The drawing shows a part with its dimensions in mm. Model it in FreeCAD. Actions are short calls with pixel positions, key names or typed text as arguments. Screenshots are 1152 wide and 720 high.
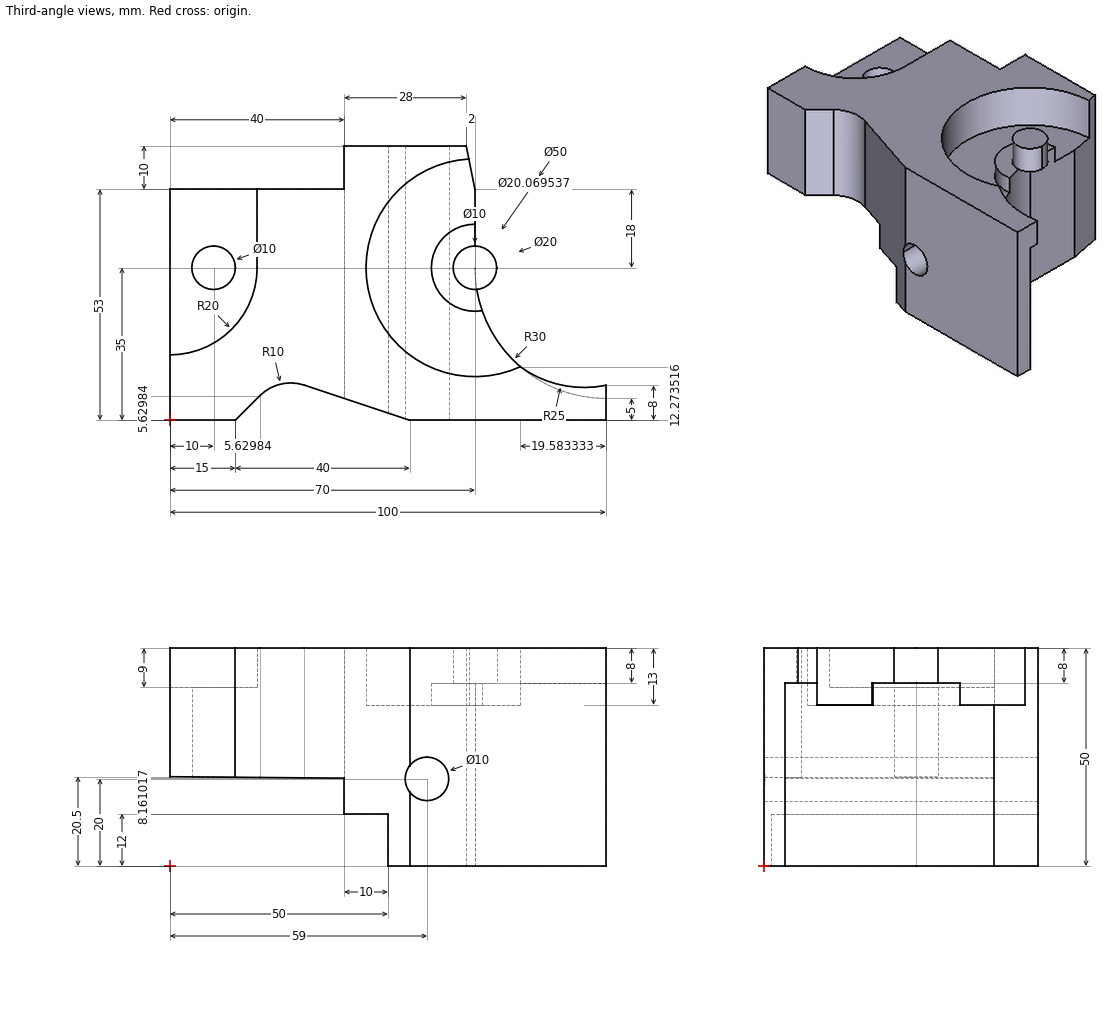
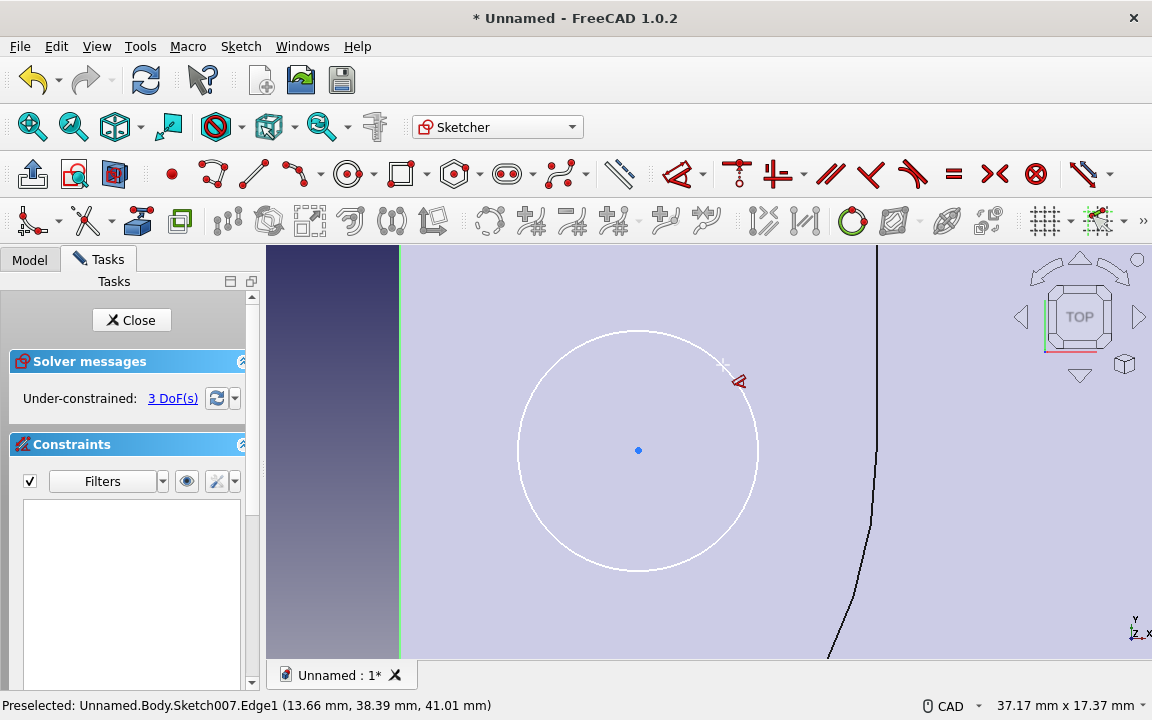
click(723, 366)
click(746, 343)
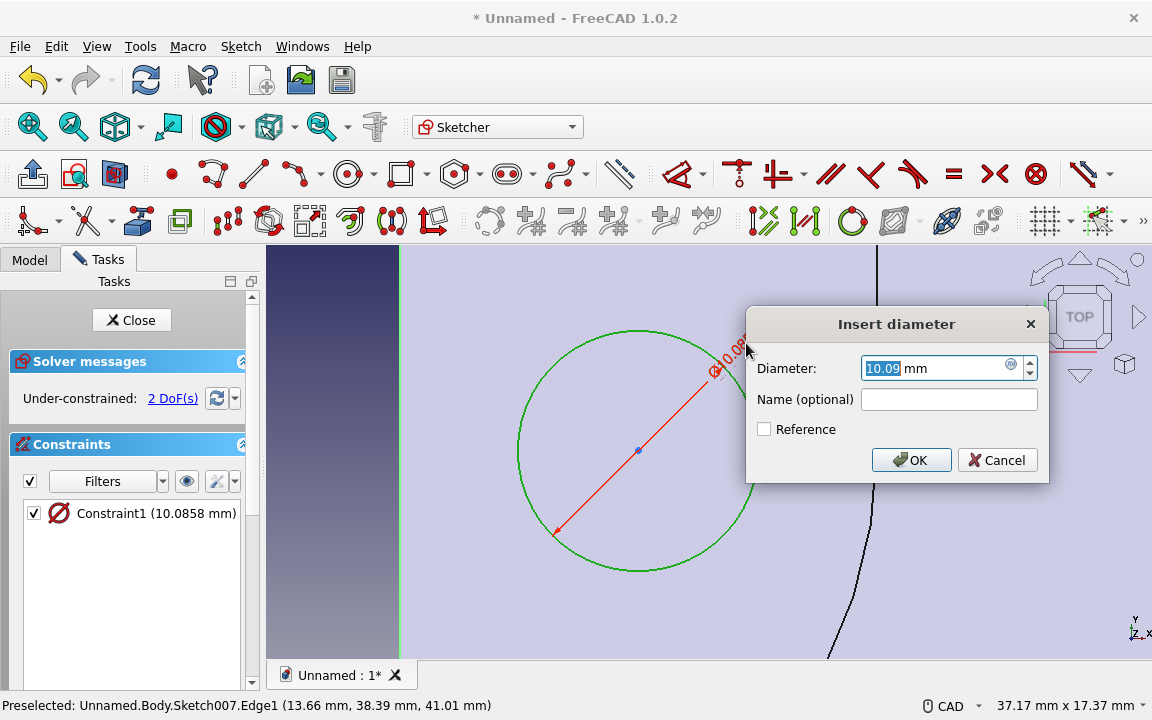
text(10)
key(Return)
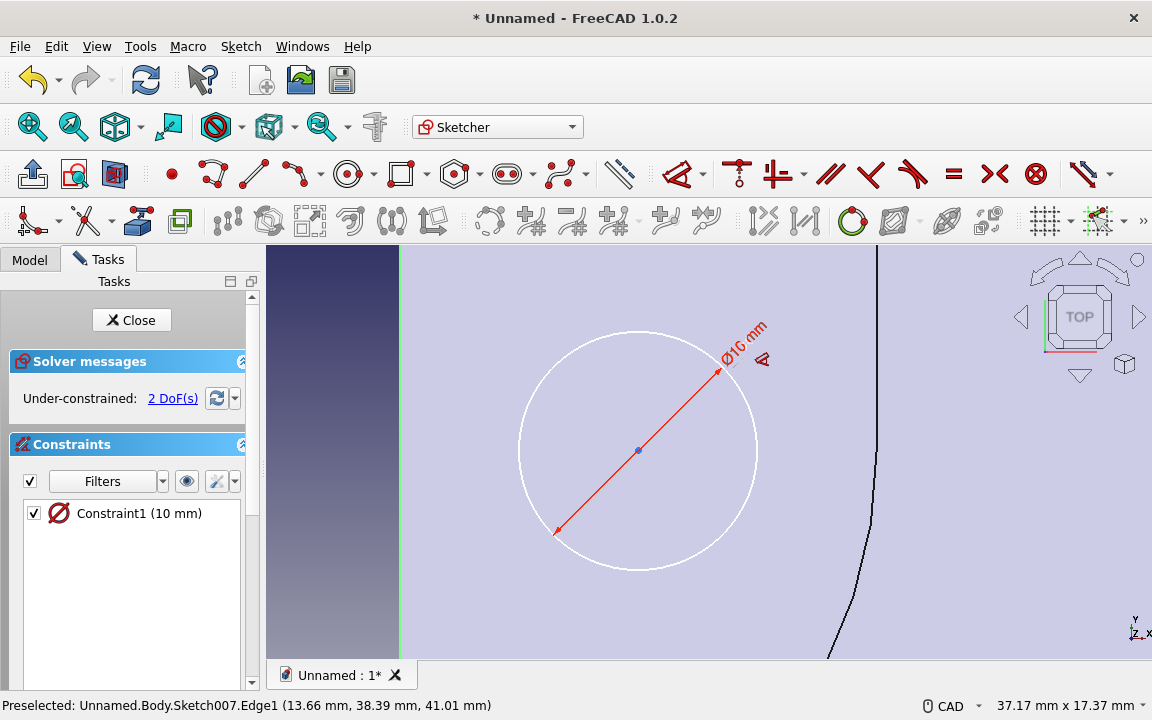
click(638, 451)
click(464, 417)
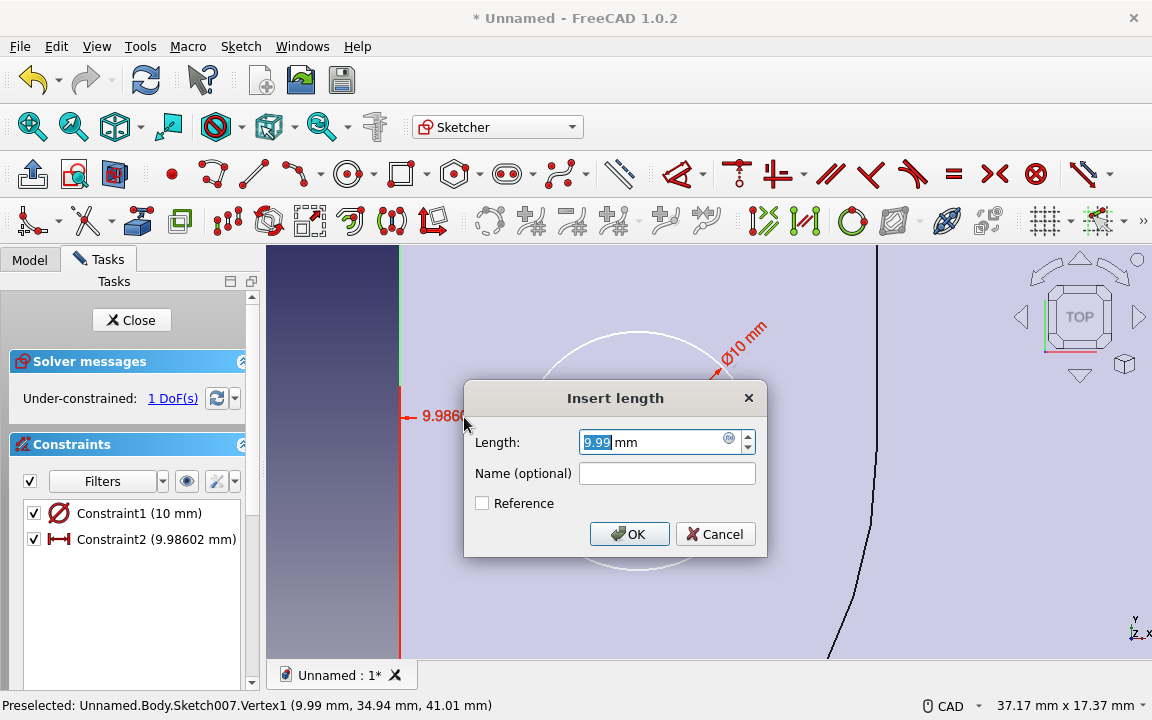
text(10)
key(Return)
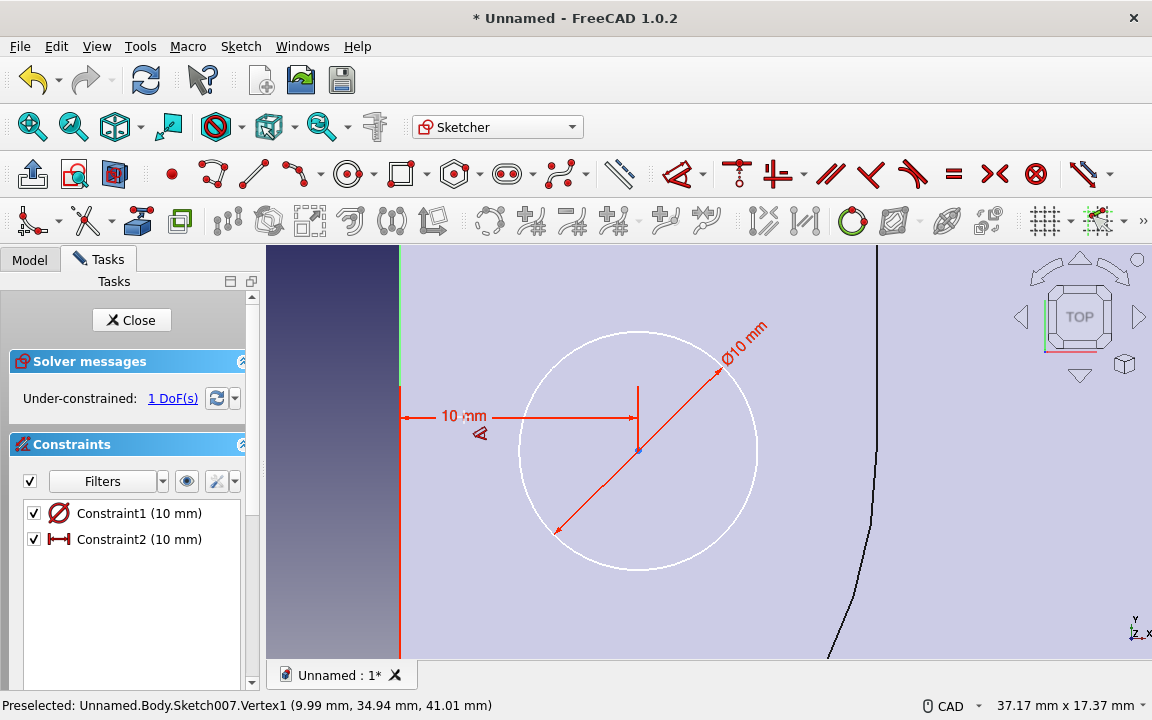
click(638, 451)
click(366, 541)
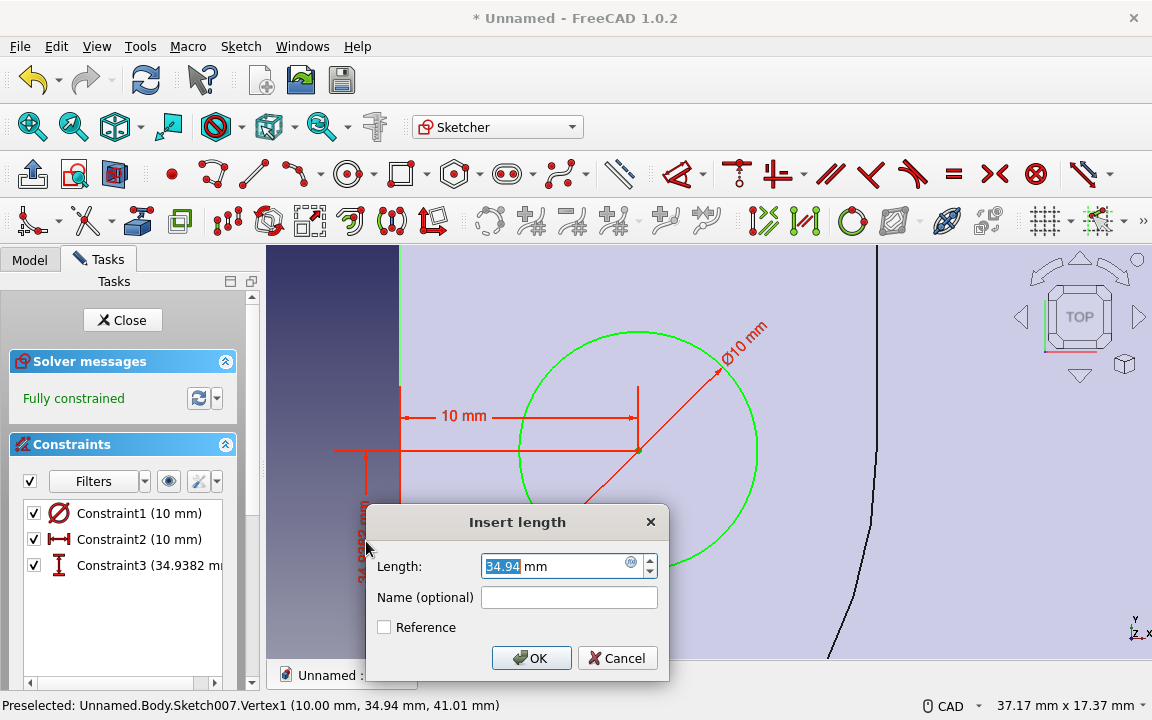
text(35)
key(Return)
key(Escape)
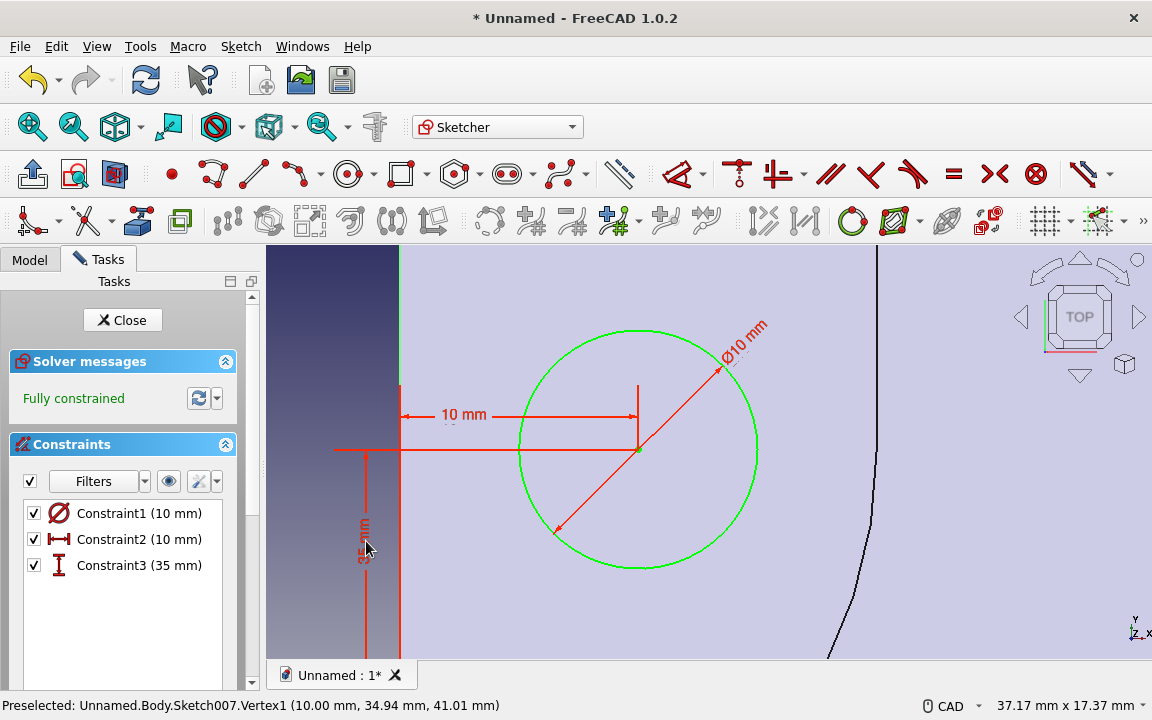
click(123, 320)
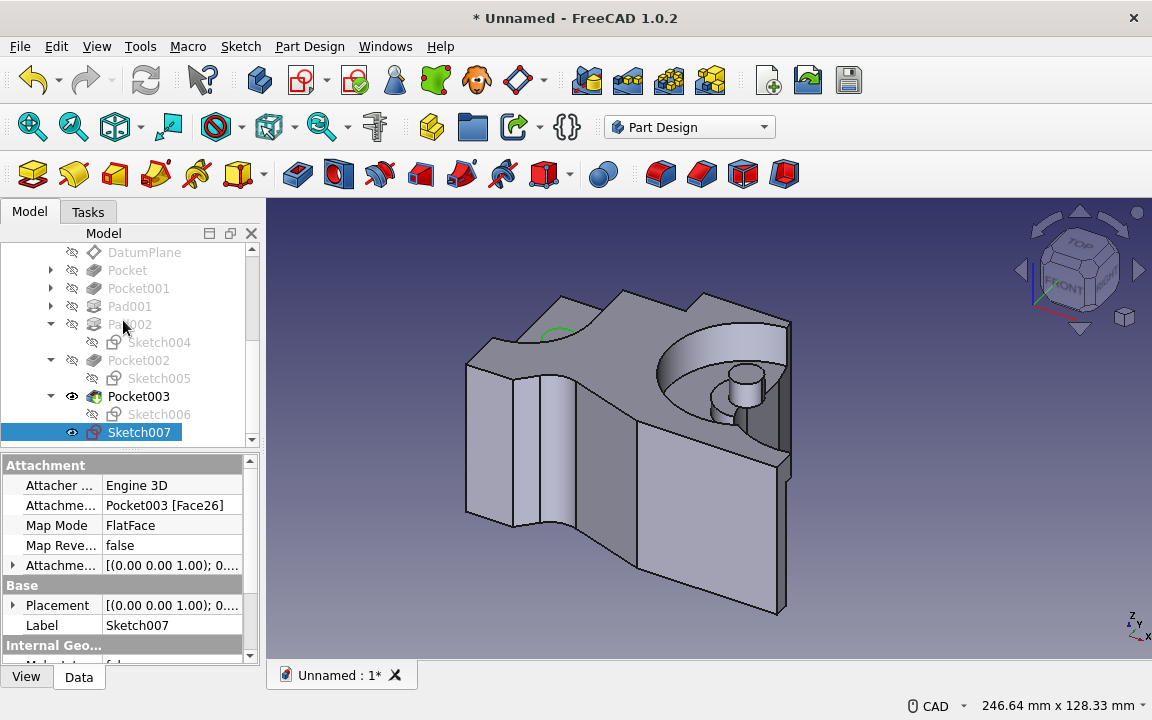
click(298, 174)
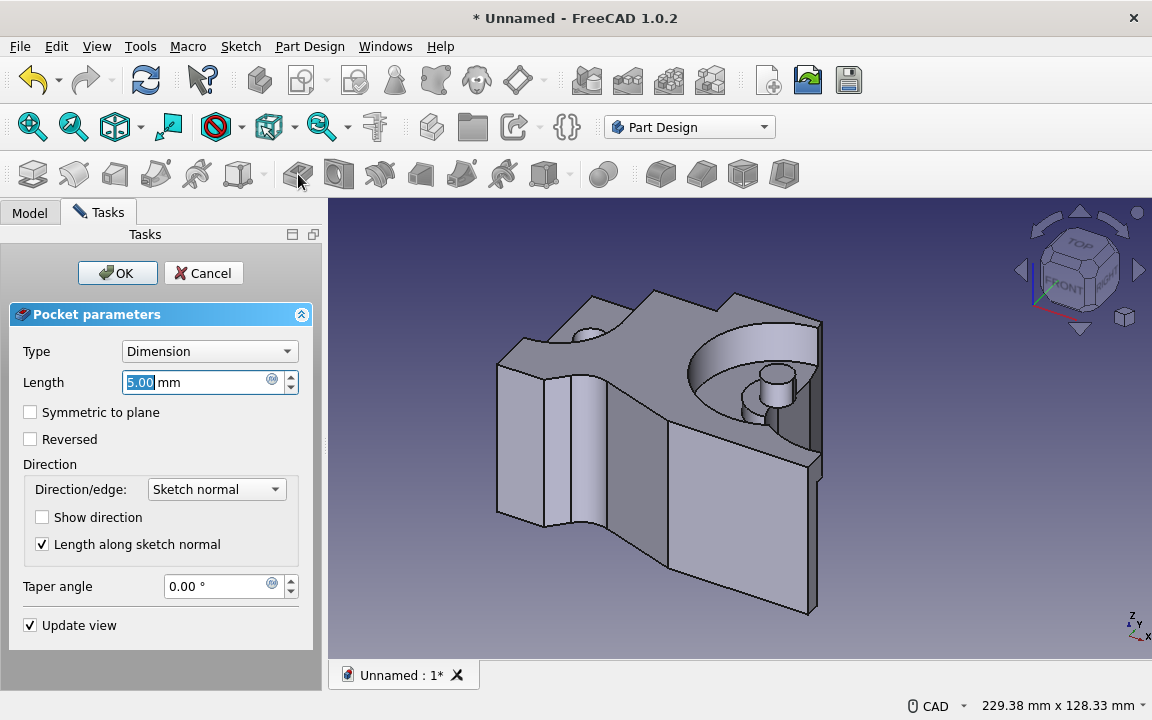
click(210, 352)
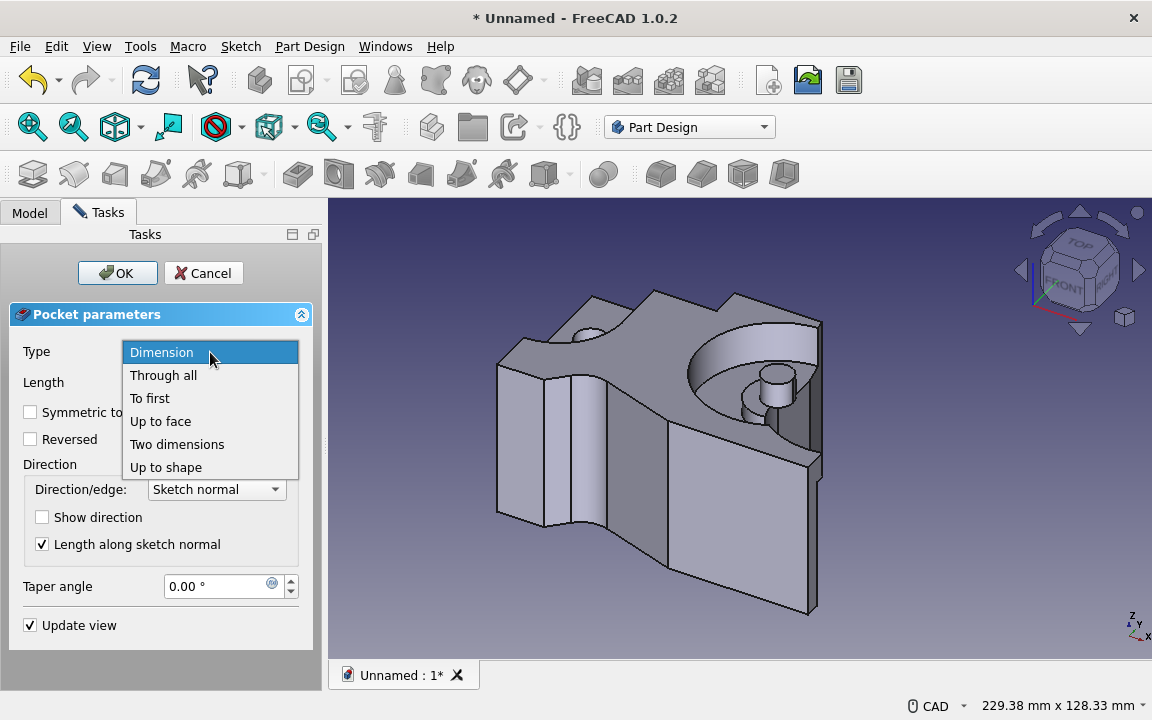
click(208, 376)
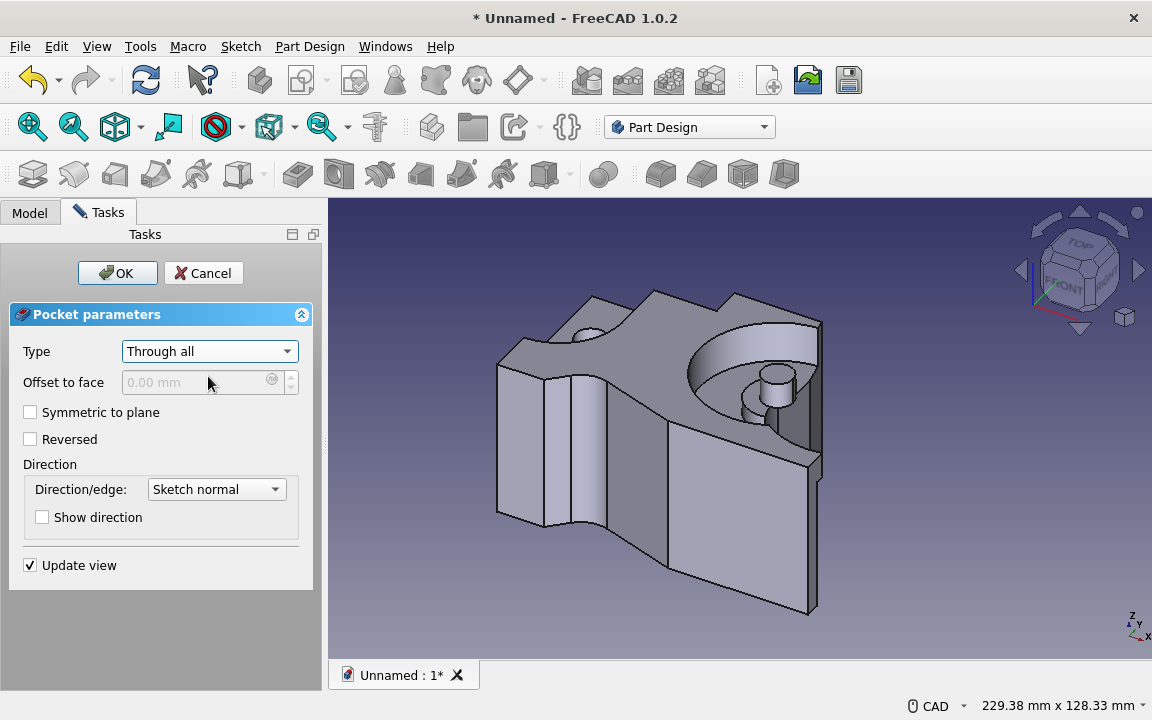
click(118, 273)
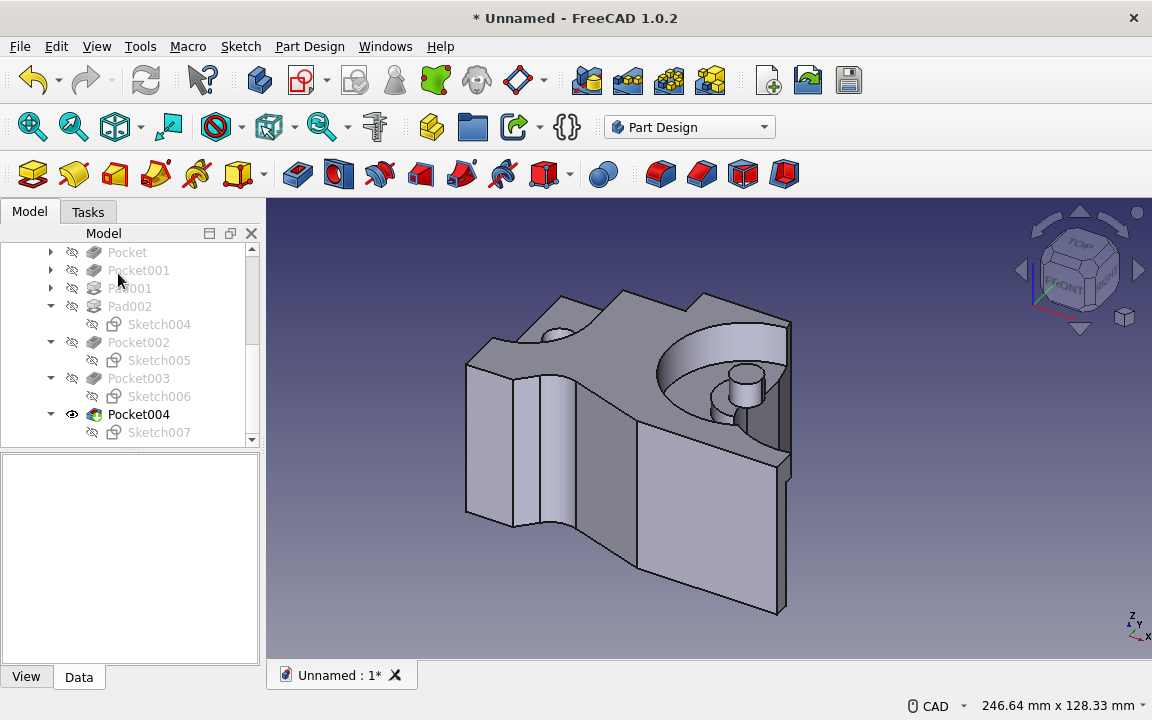
key(4)